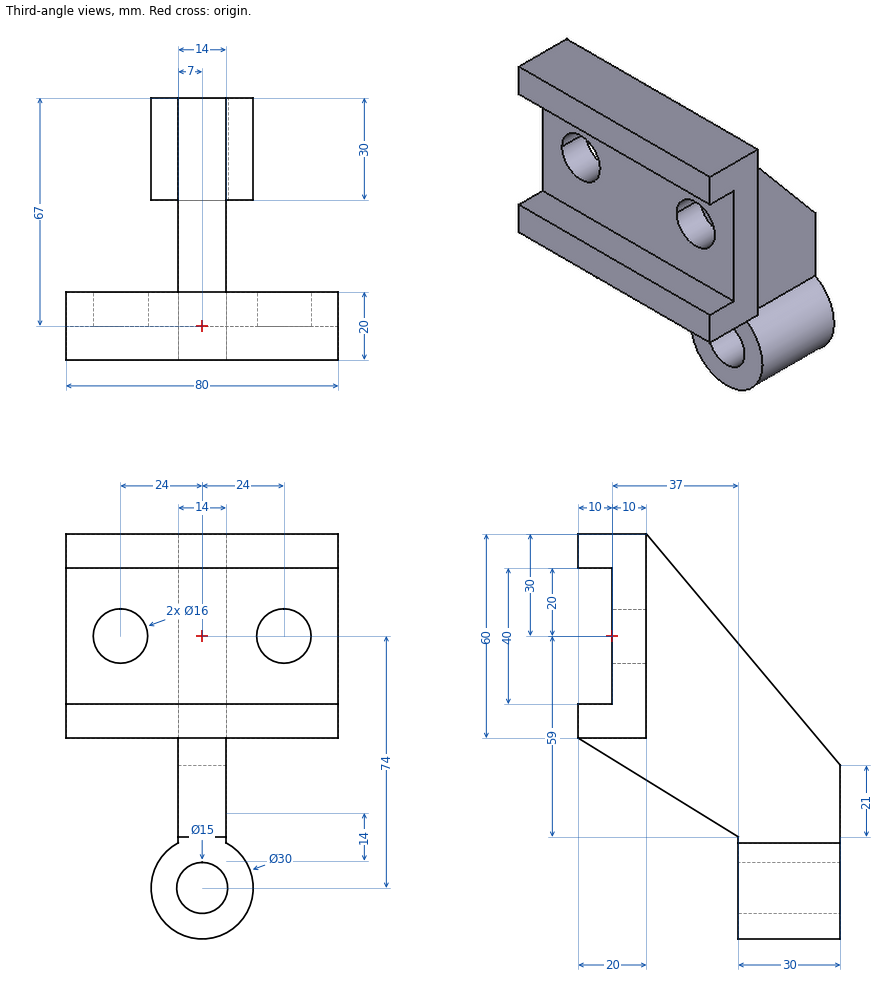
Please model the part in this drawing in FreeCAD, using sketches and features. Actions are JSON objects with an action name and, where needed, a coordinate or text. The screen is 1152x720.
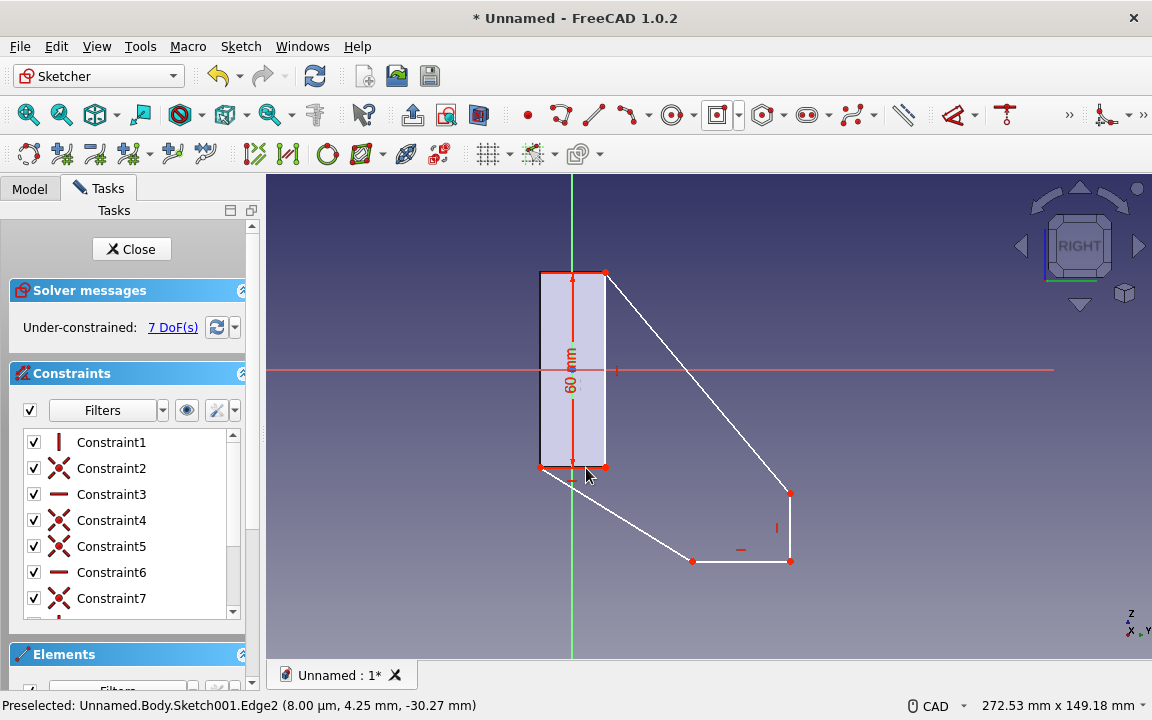
{"action": "key", "text": "l"}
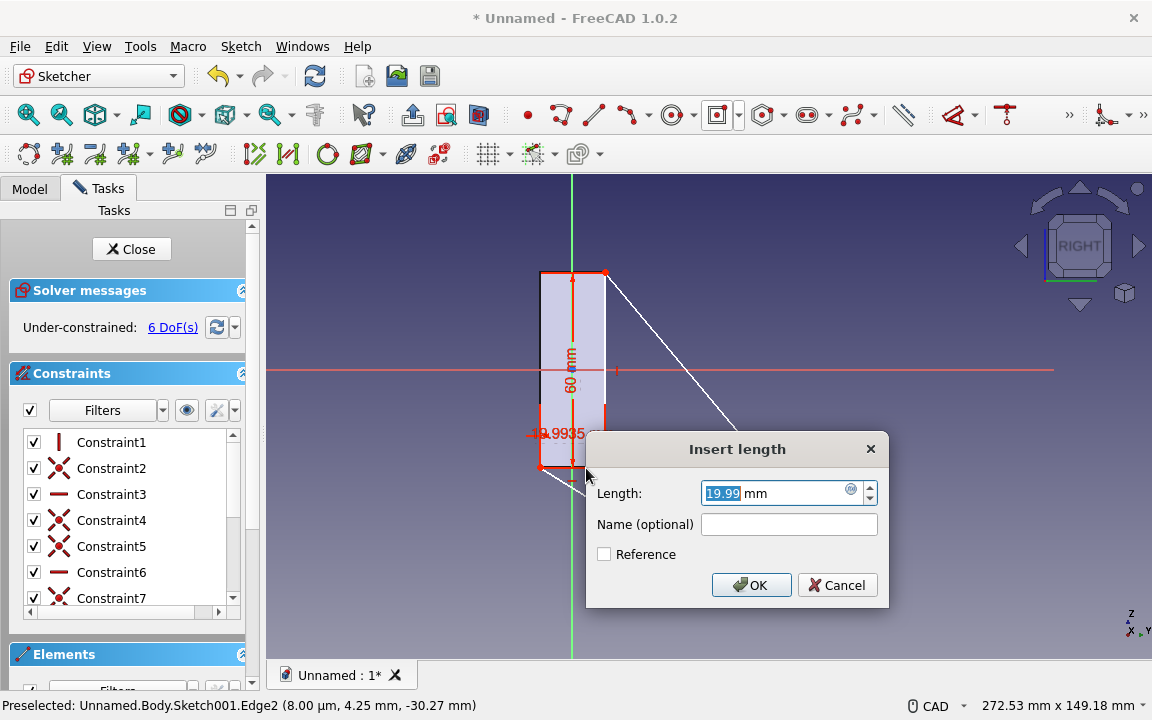
{"action": "type", "text": "20"}
{"action": "key", "text": "Return"}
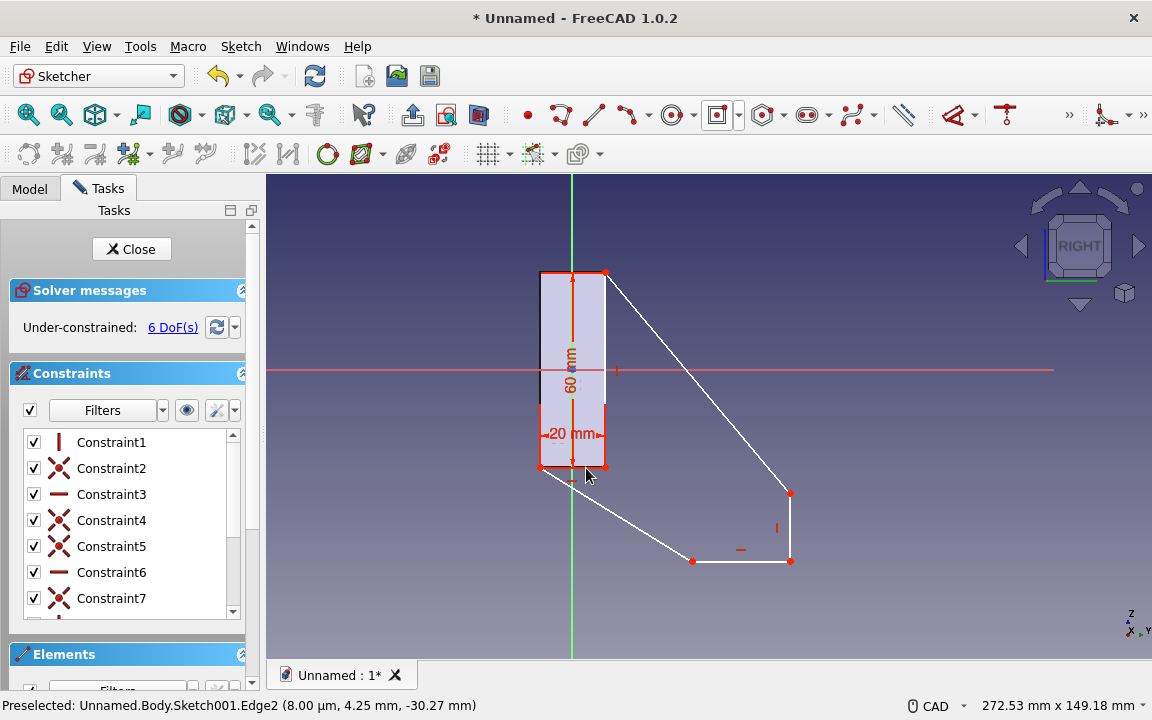
{"action": "left_click", "coordinate": [721, 562]}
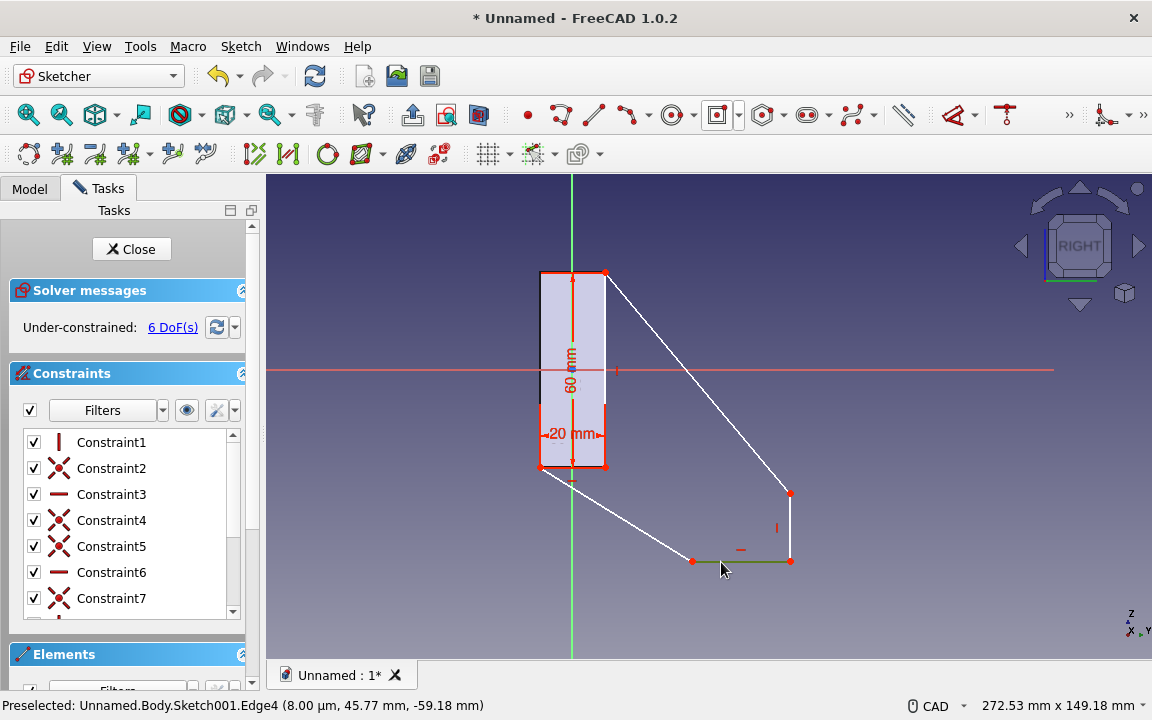
{"action": "key", "text": "l"}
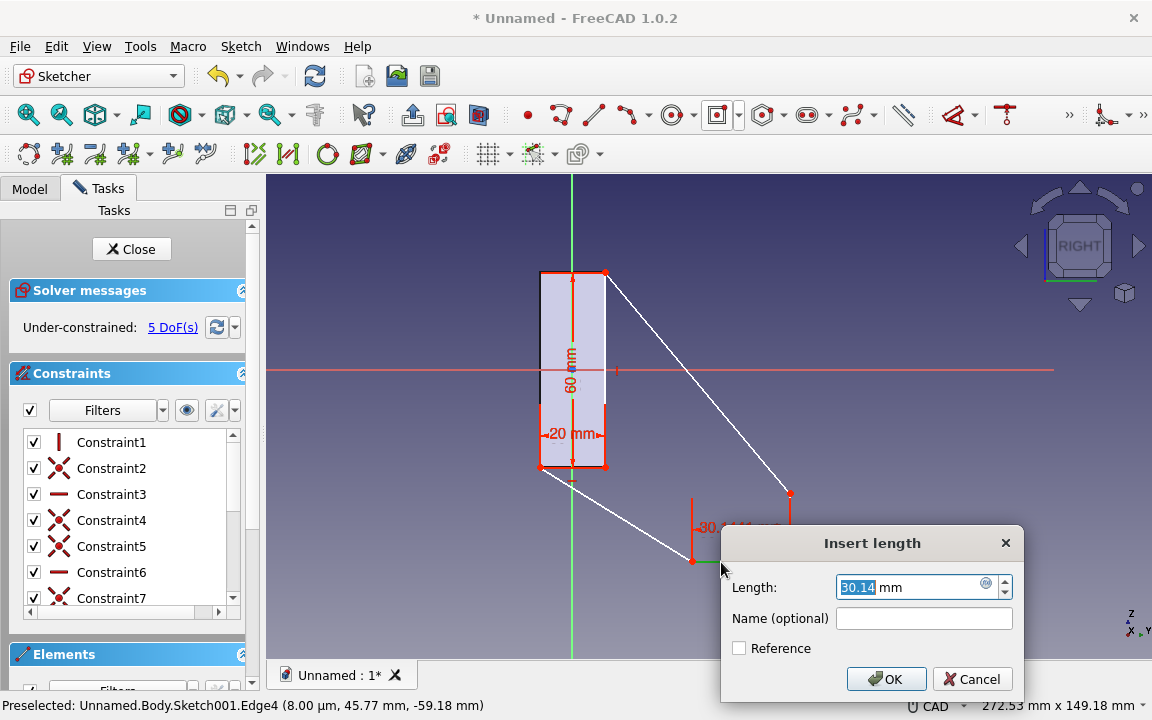
{"action": "type", "text": "30"}
{"action": "key", "text": "Return"}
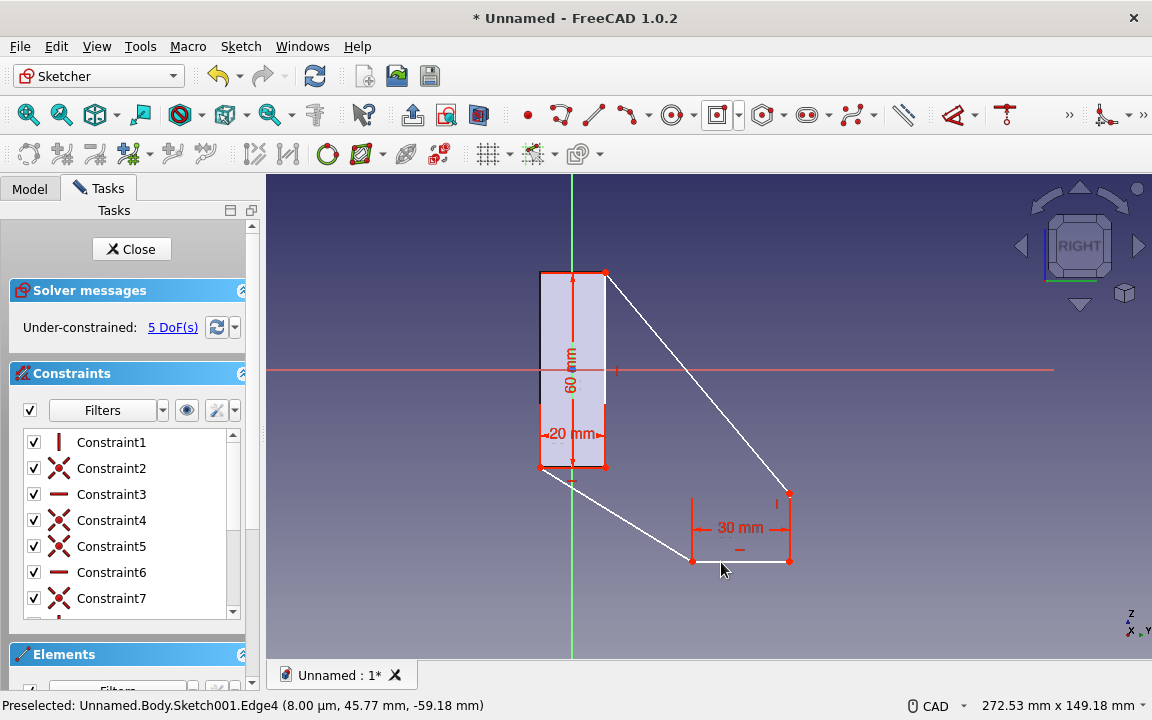
{"action": "left_click", "coordinate": [790, 542]}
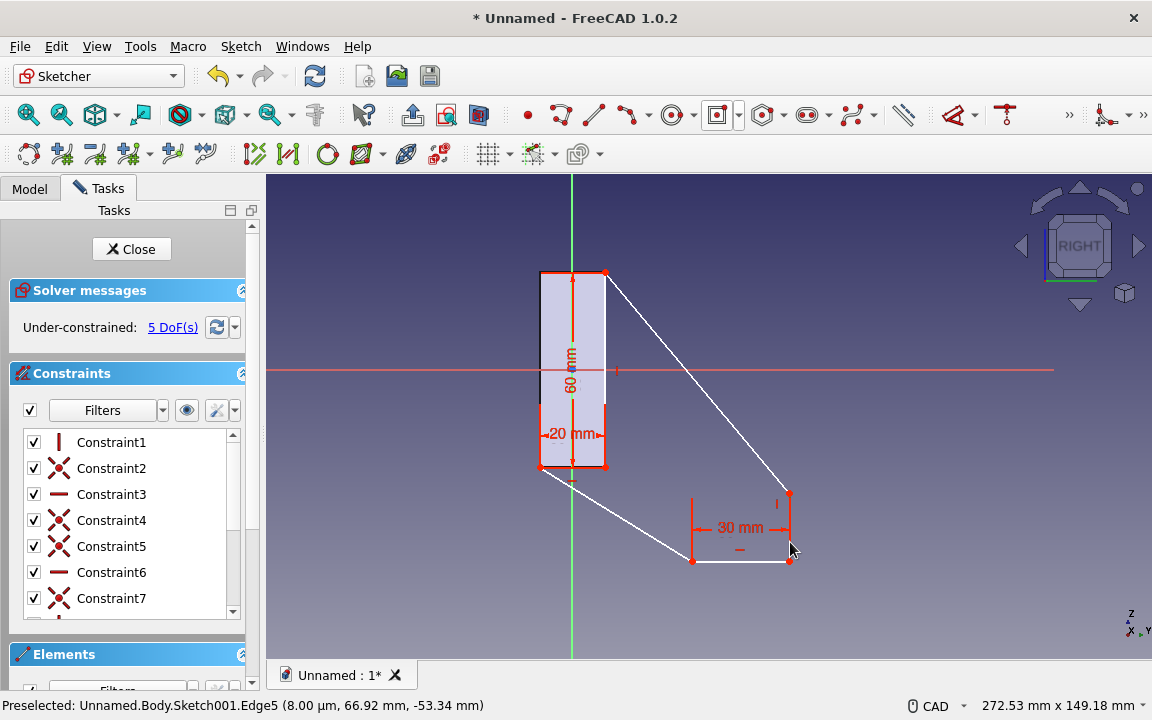
{"action": "left_click", "coordinate": [974, 116]}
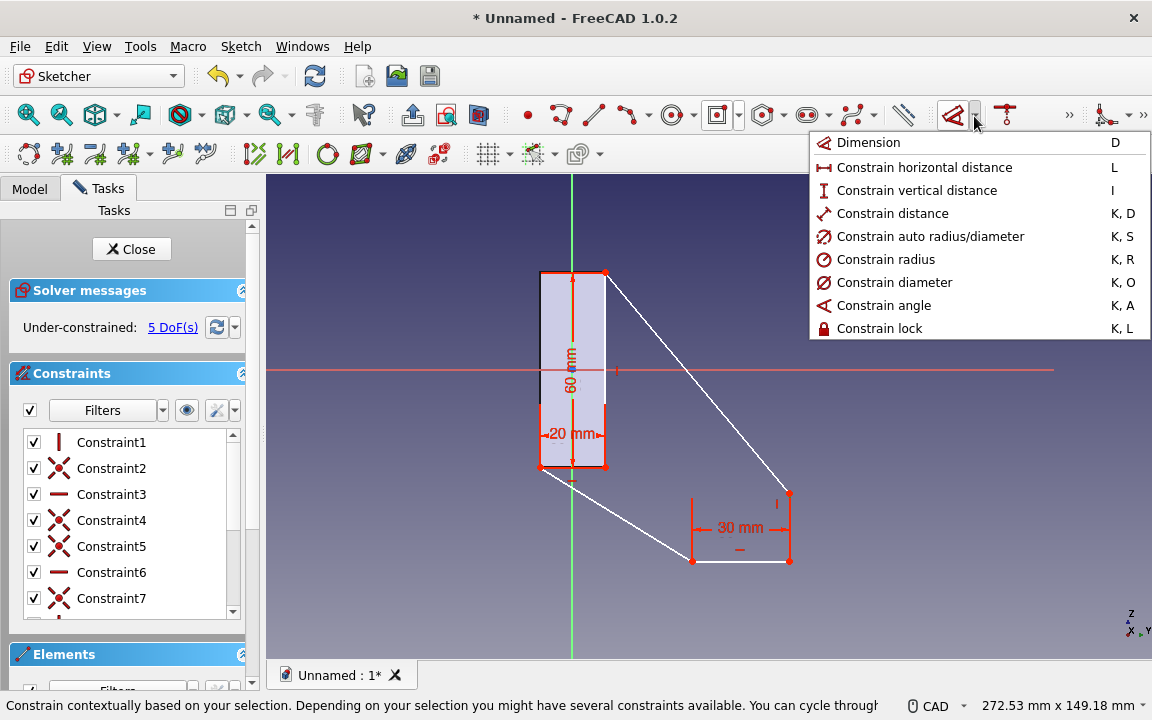
{"action": "left_click", "coordinate": [980, 190]}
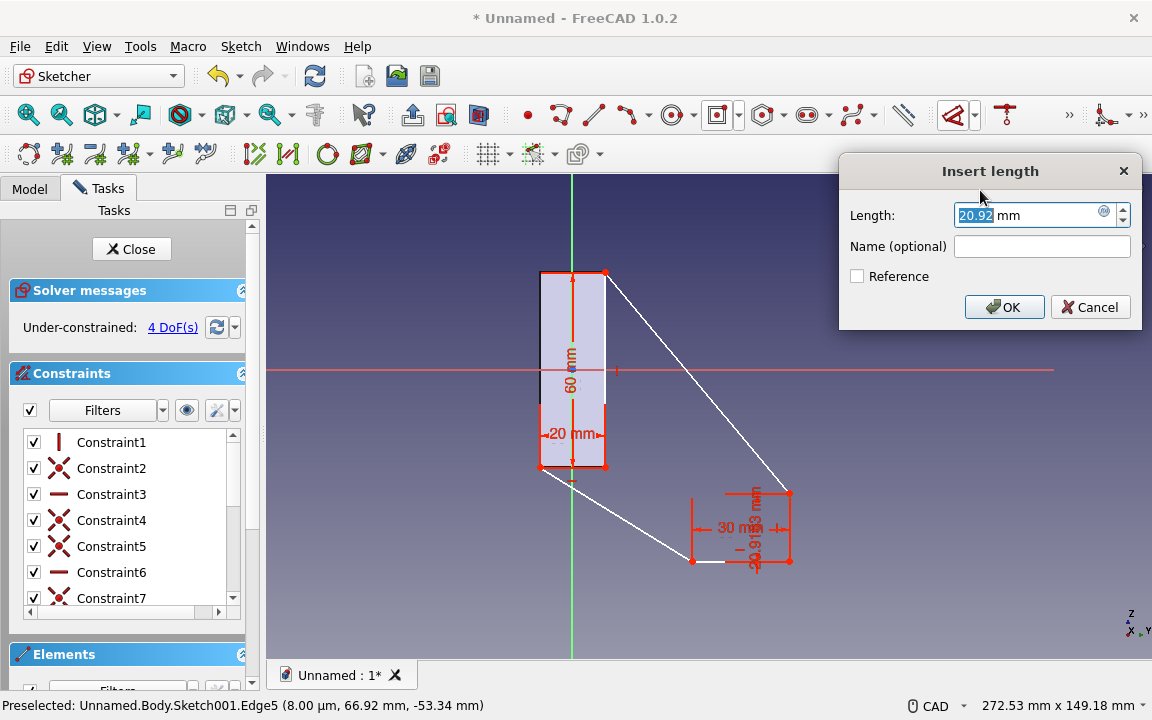
{"action": "type", "text": "21"}
{"action": "key", "text": "Return"}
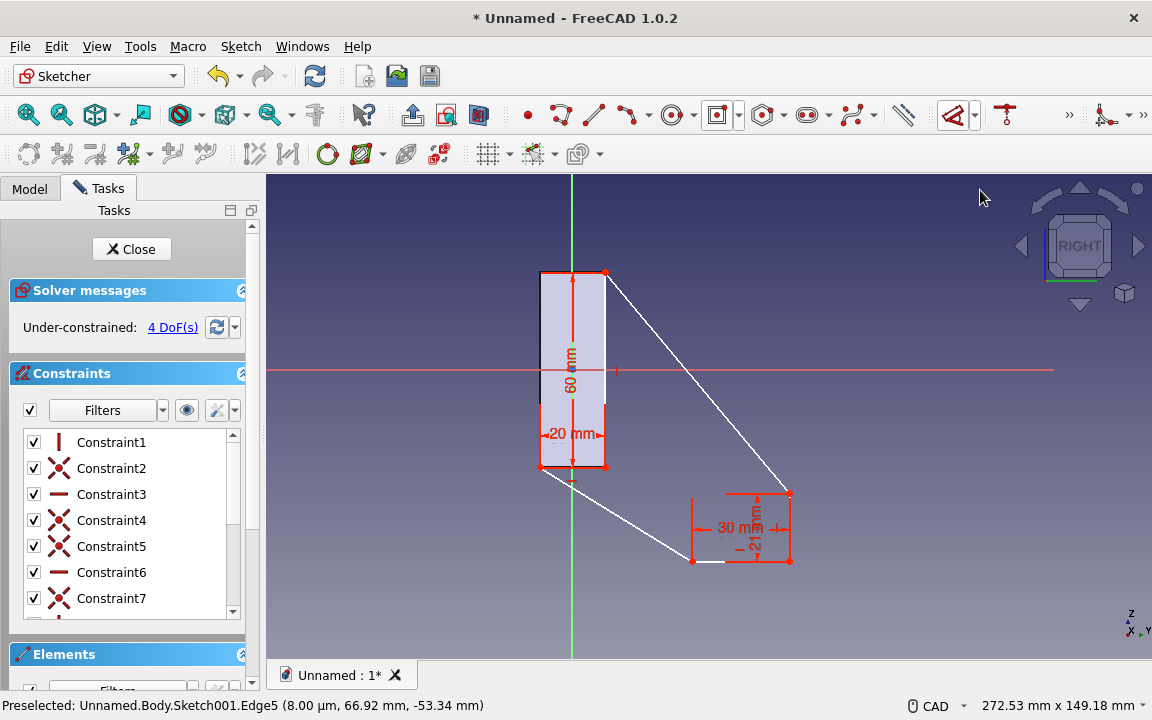
{"action": "left_click", "coordinate": [605, 273]}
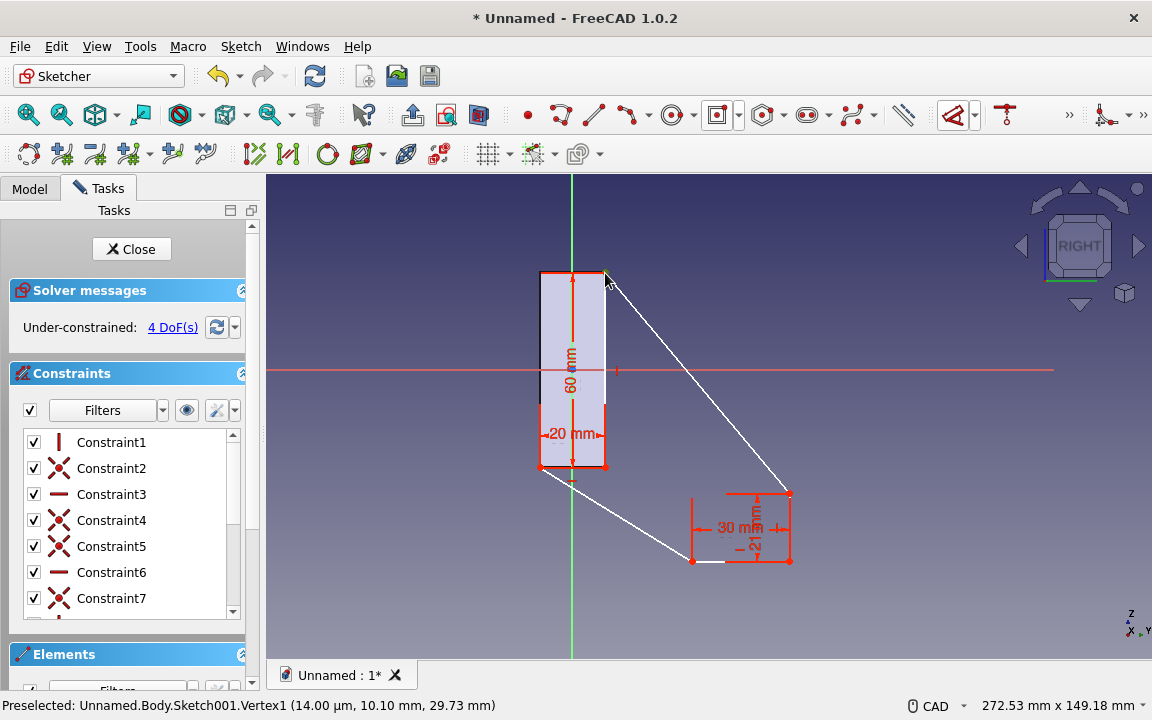
{"action": "left_click", "coordinate": [974, 116]}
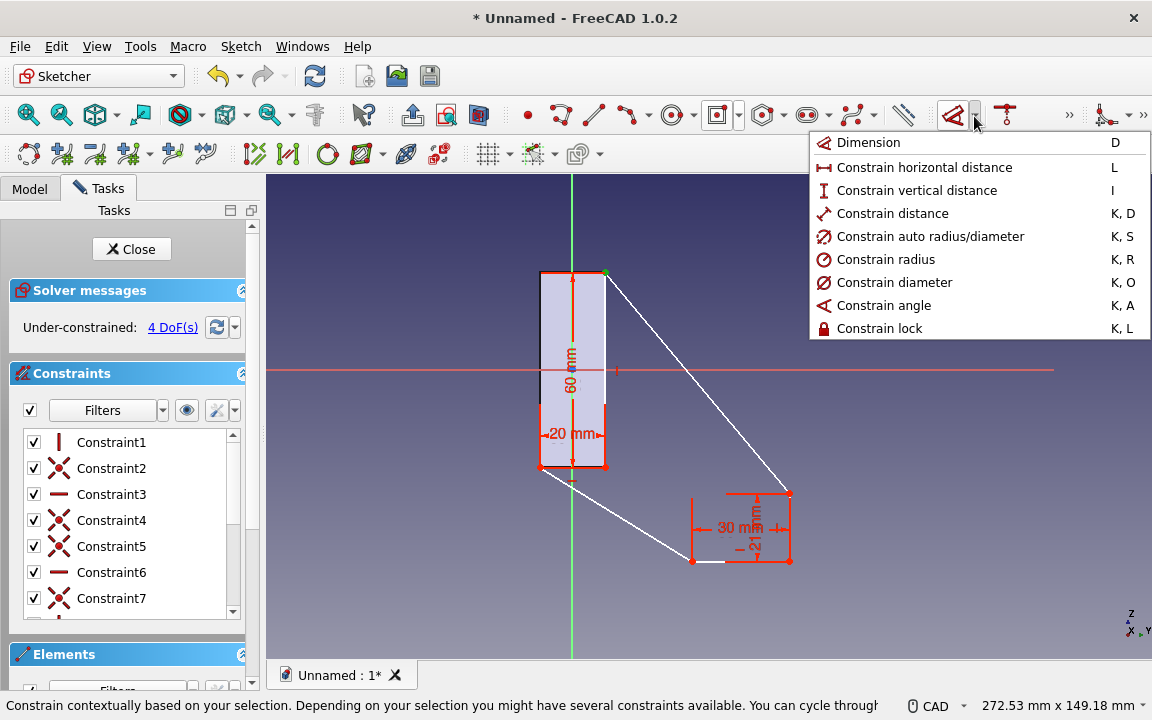
{"action": "left_click", "coordinate": [980, 168]}